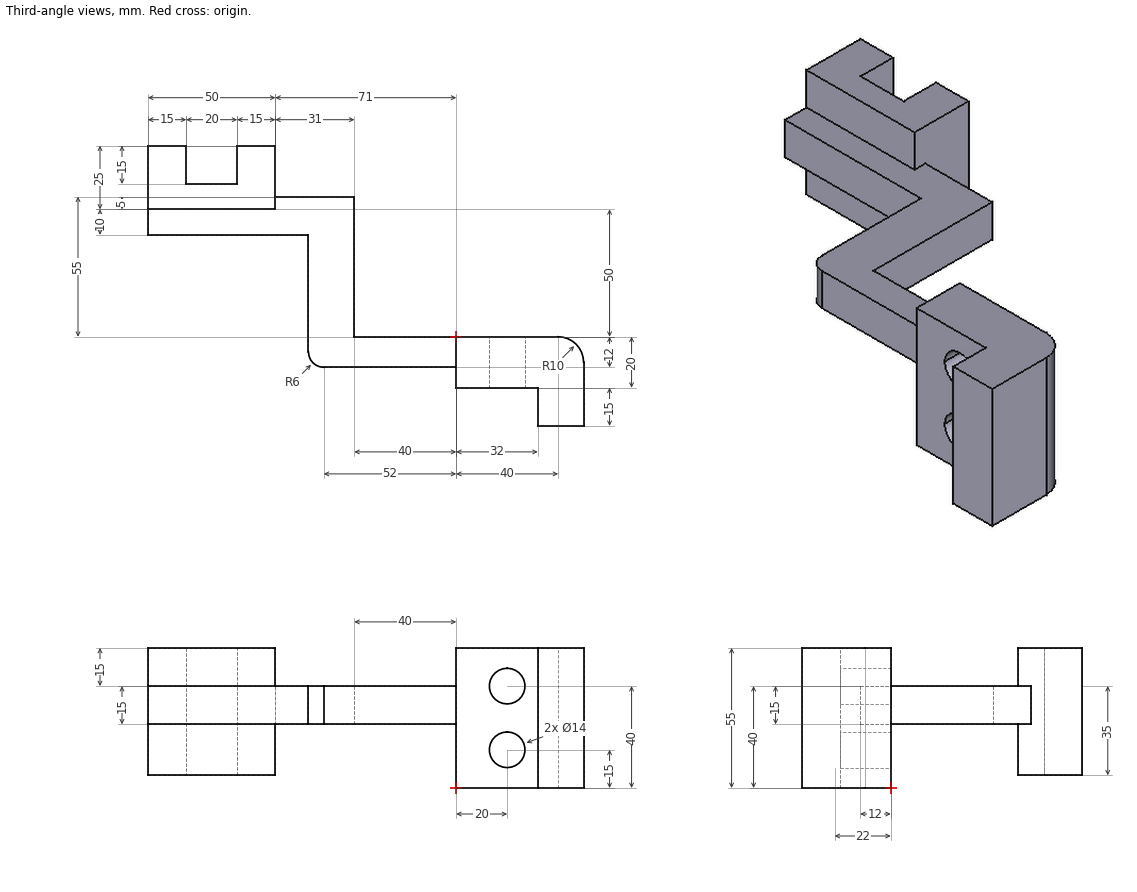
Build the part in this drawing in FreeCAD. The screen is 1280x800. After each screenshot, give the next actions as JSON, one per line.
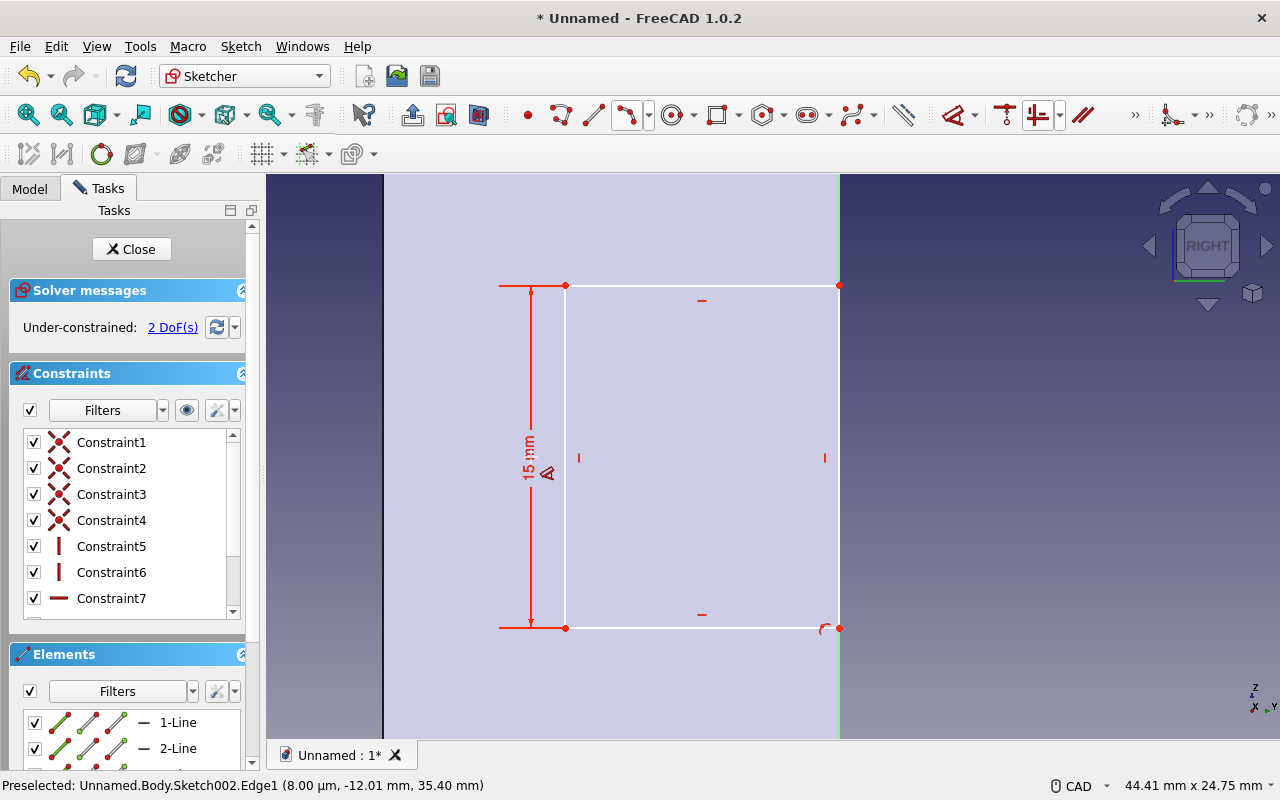
{"action": "left_click", "coordinate": [647, 628]}
{"action": "left_click", "coordinate": [702, 662]}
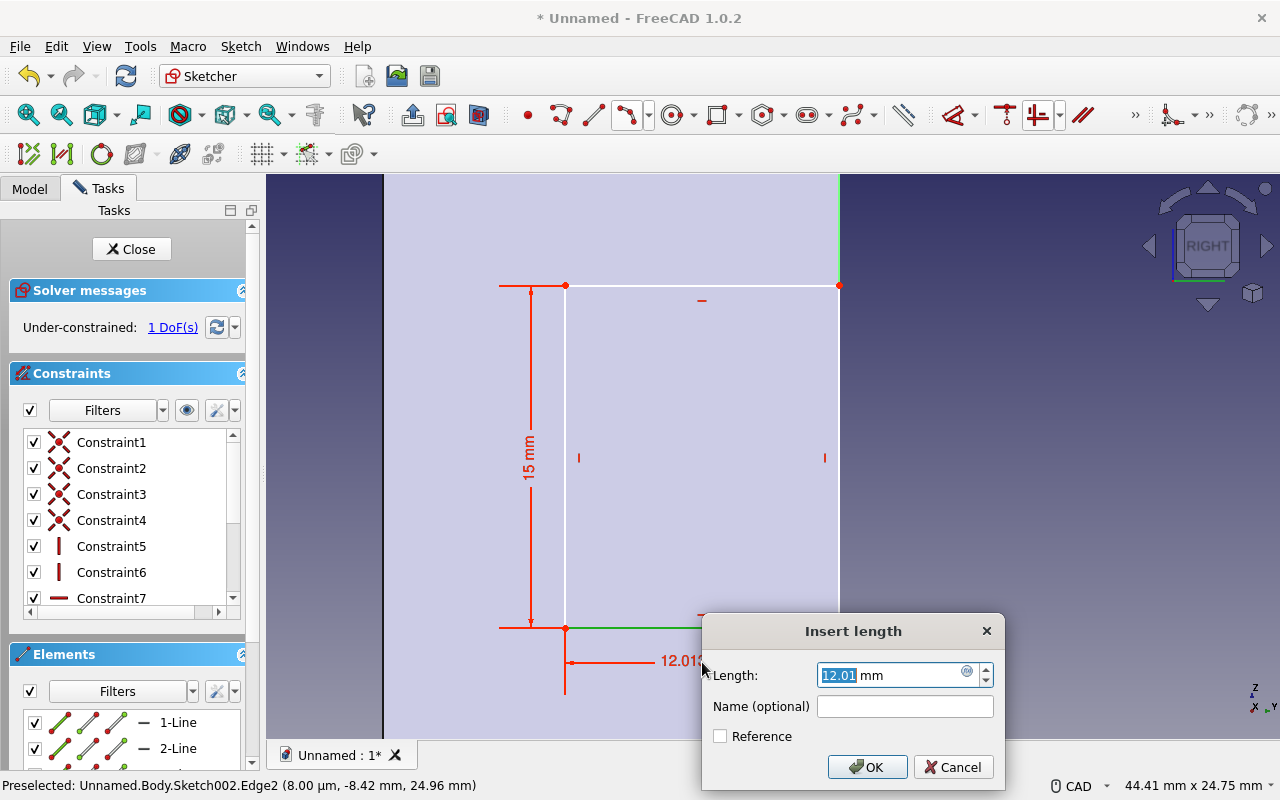
{"action": "type", "text": "12"}
{"action": "key", "text": "Return"}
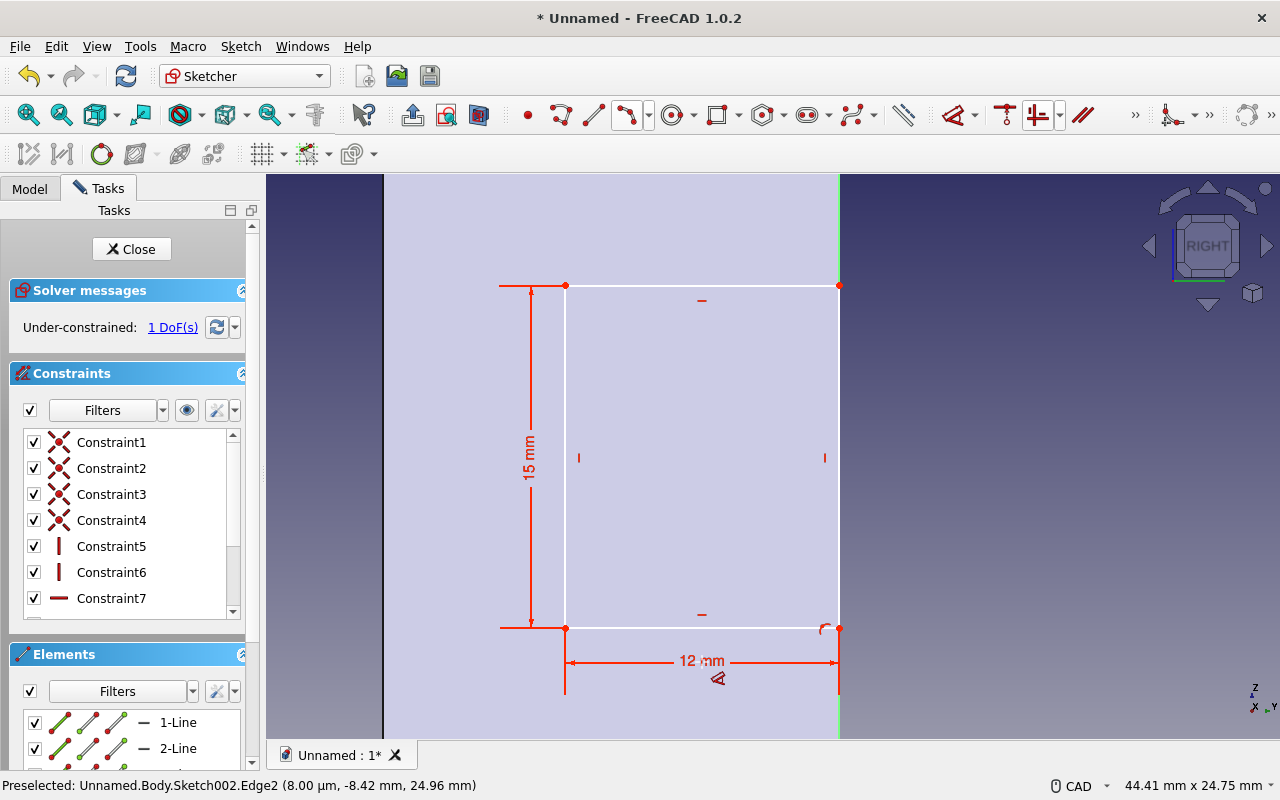
{"action": "left_click", "coordinate": [565, 286]}
{"action": "left_click", "coordinate": [873, 499]}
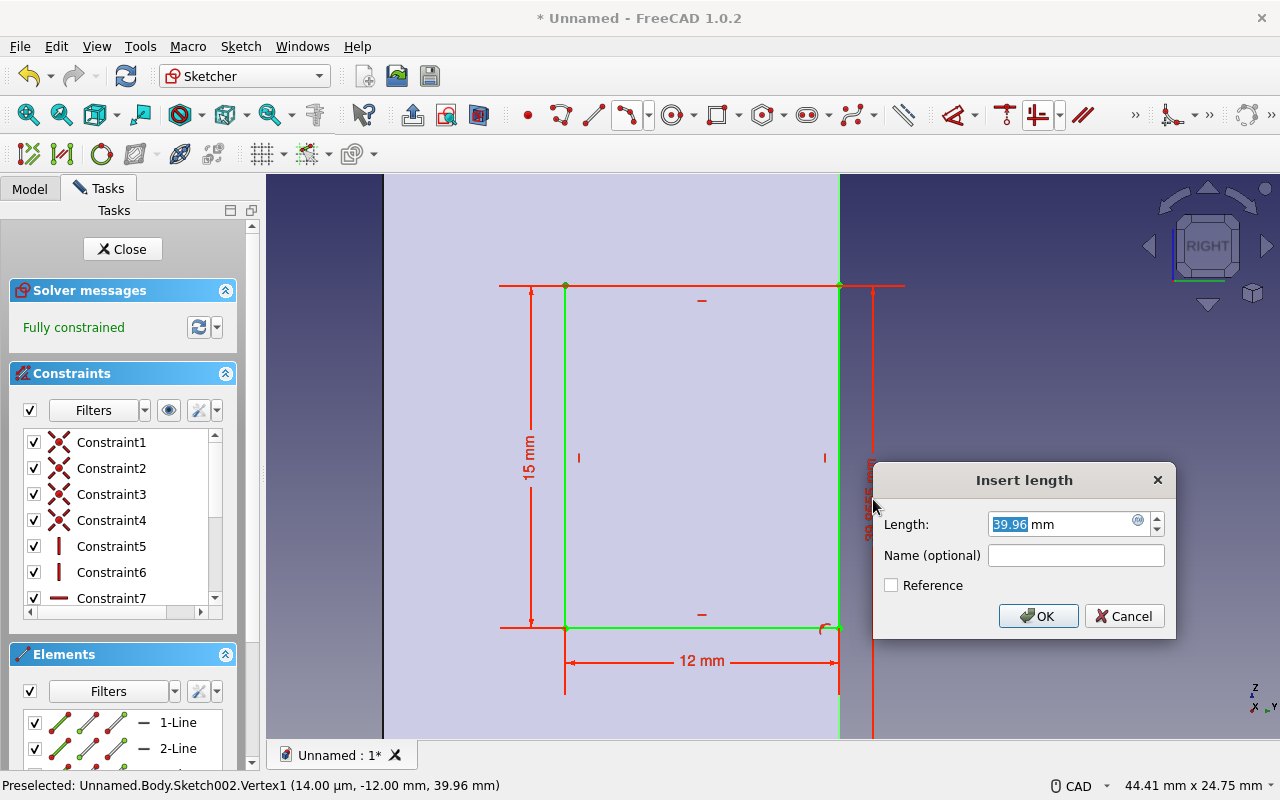
{"action": "type", "text": "40"}
{"action": "key", "text": "Return"}
{"action": "key", "text": "Escape"}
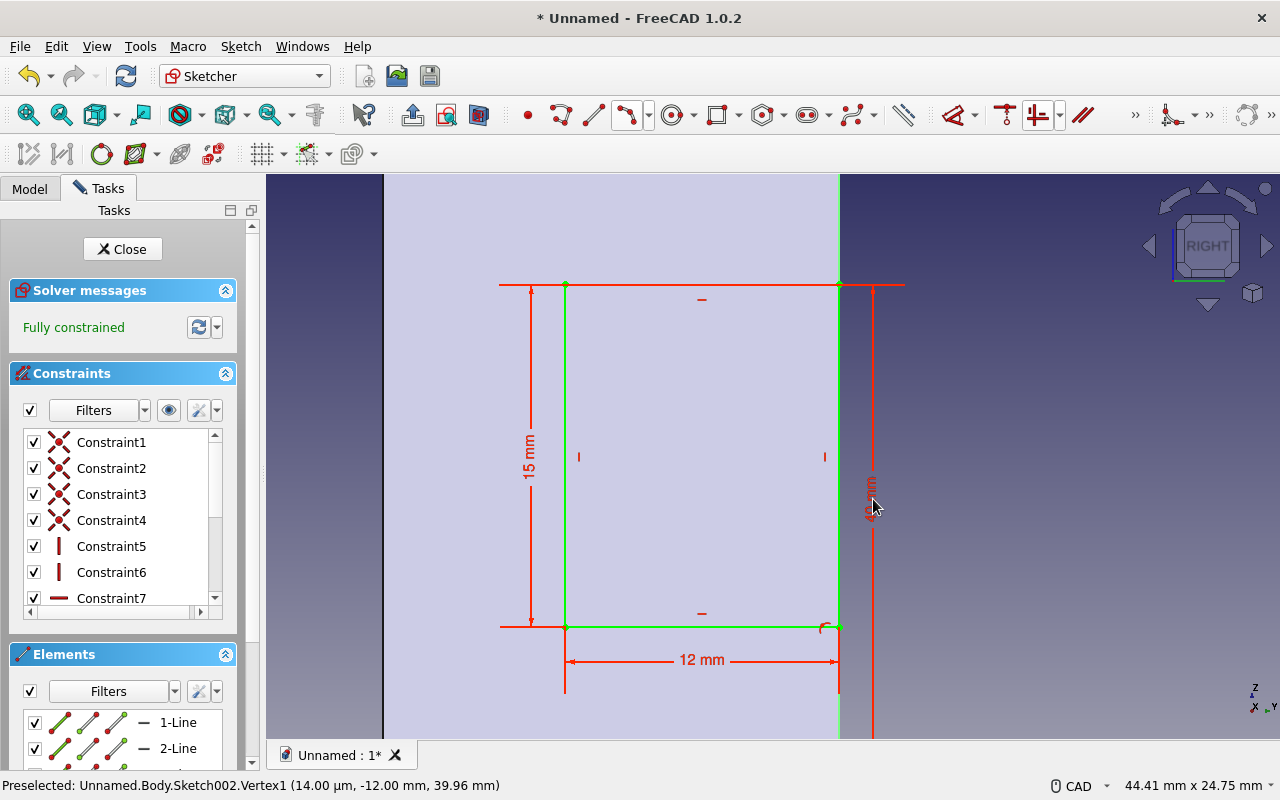
{"action": "left_click", "coordinate": [123, 249]}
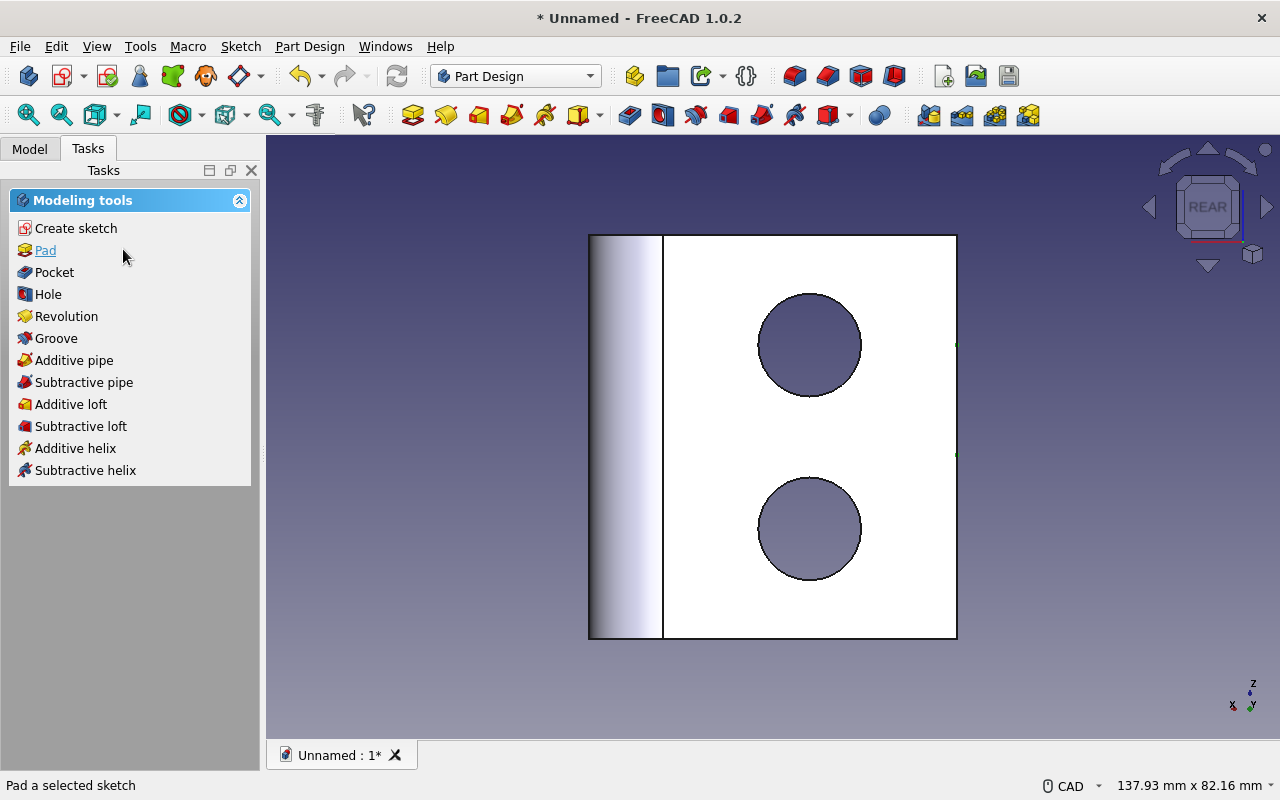
{"action": "left_click", "coordinate": [413, 116]}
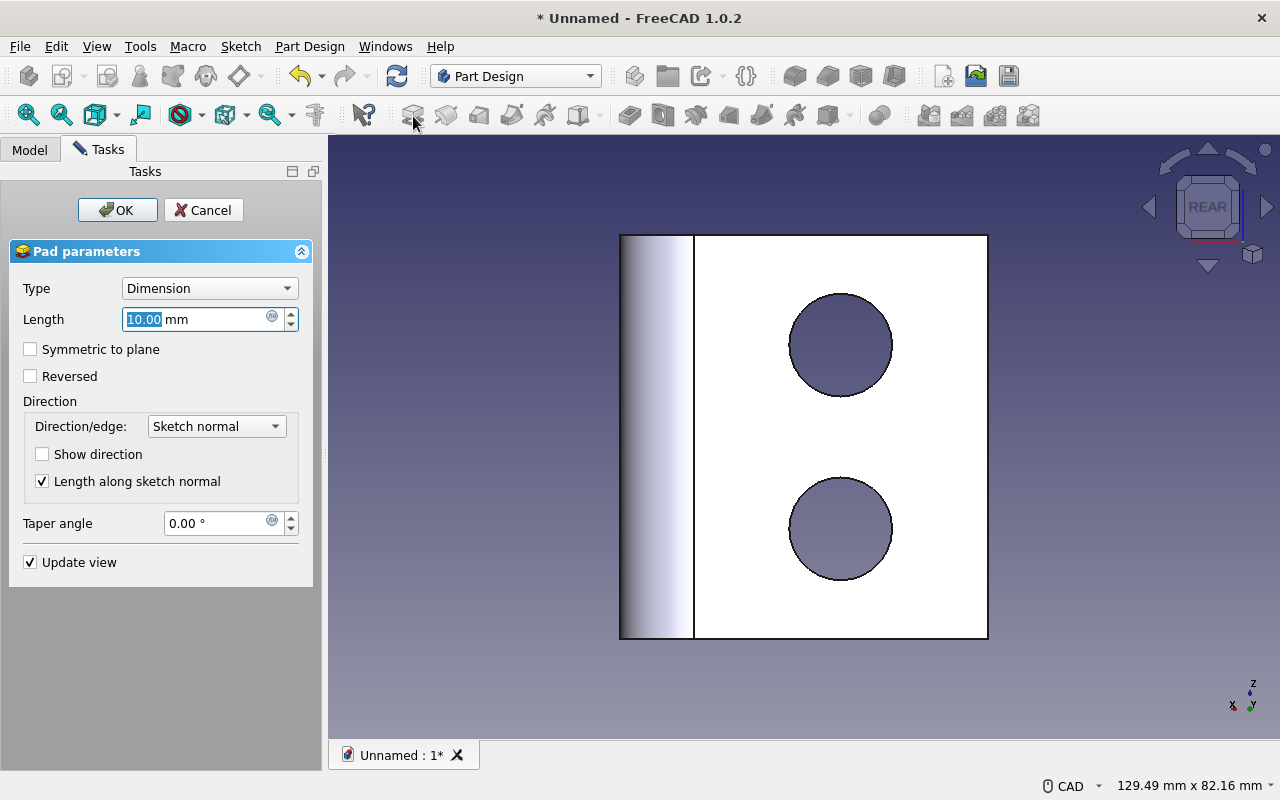
{"action": "type", "text": "40"}
{"action": "key", "text": "Tab"}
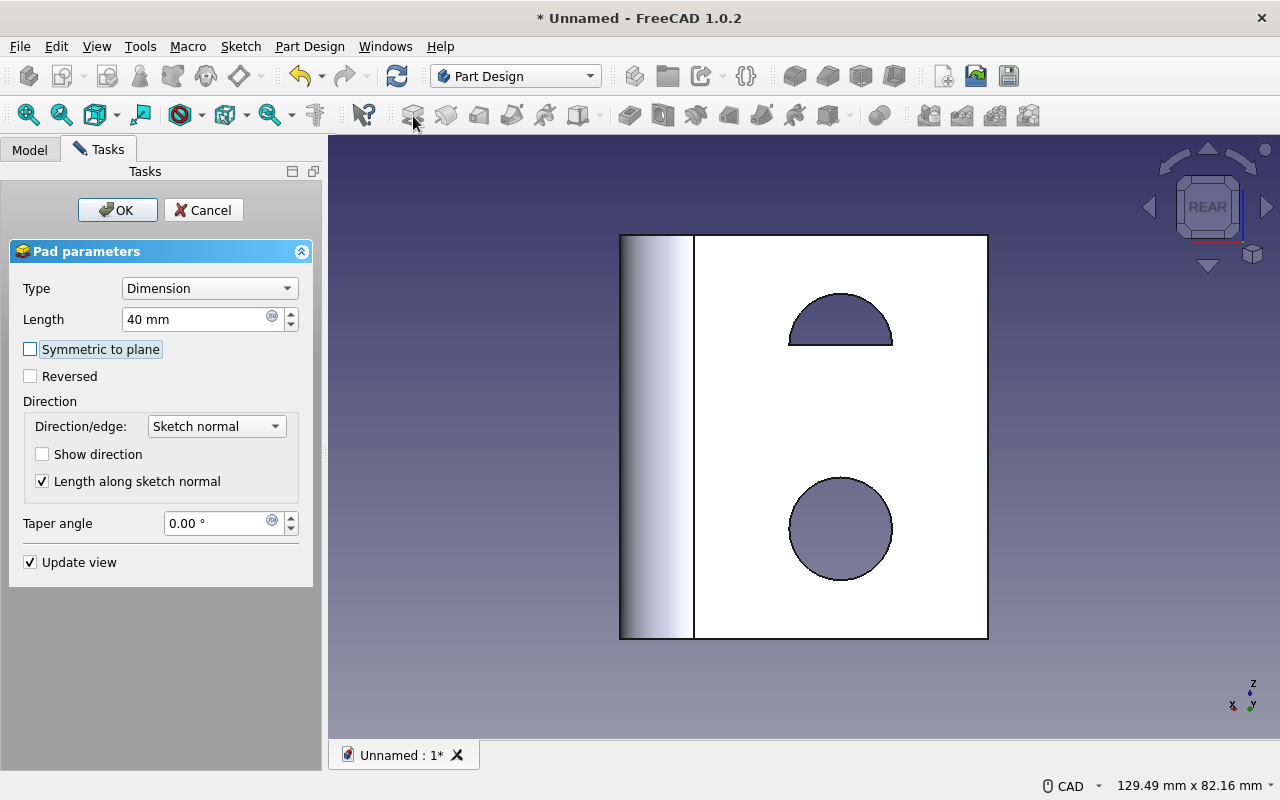
{"action": "left_click", "coordinate": [31, 376]}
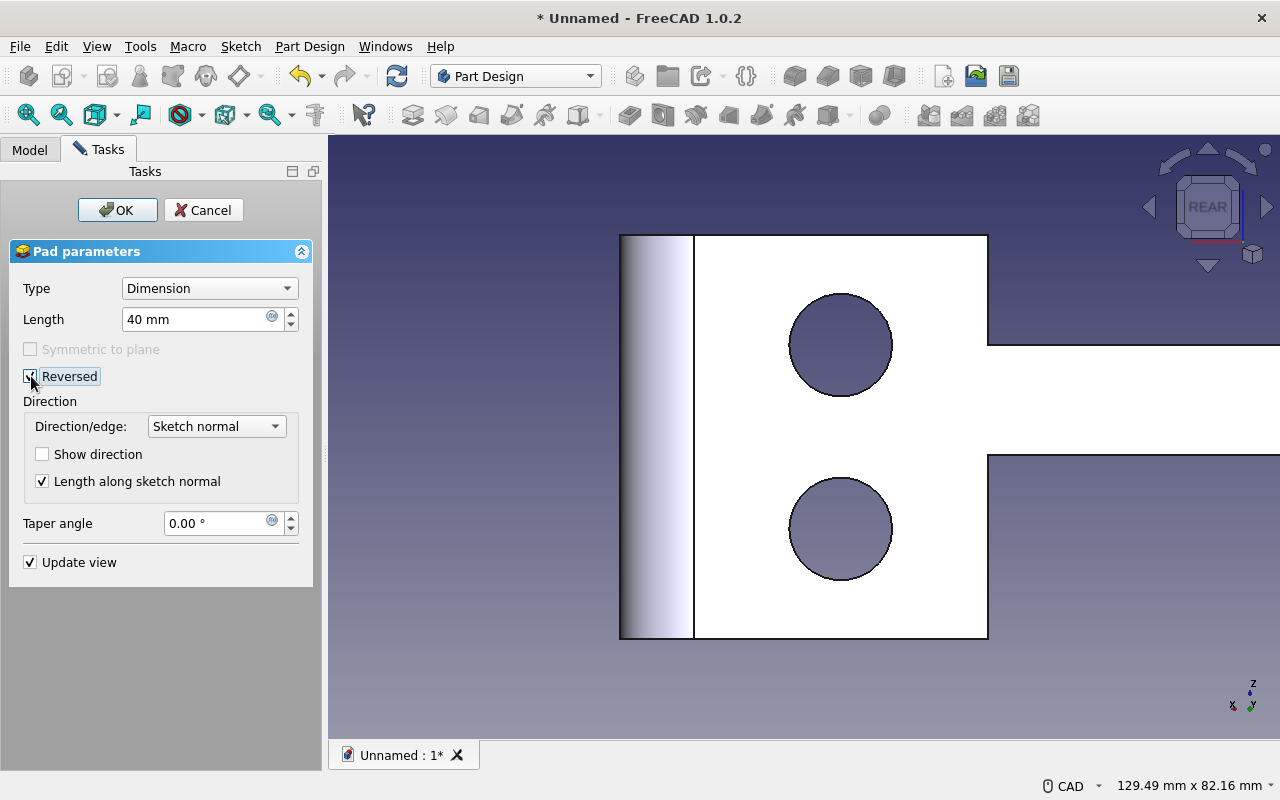
{"action": "left_click", "coordinate": [118, 210]}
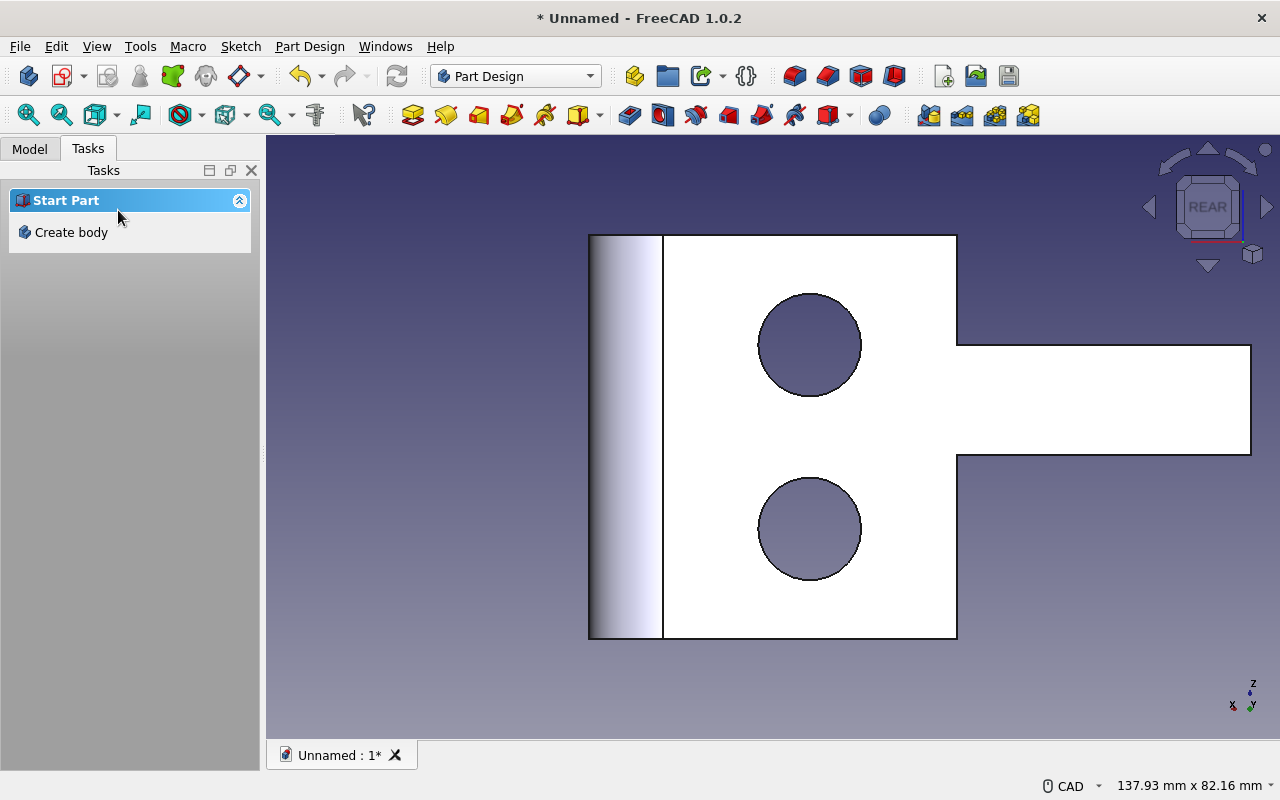
{"action": "key", "text": "0"}